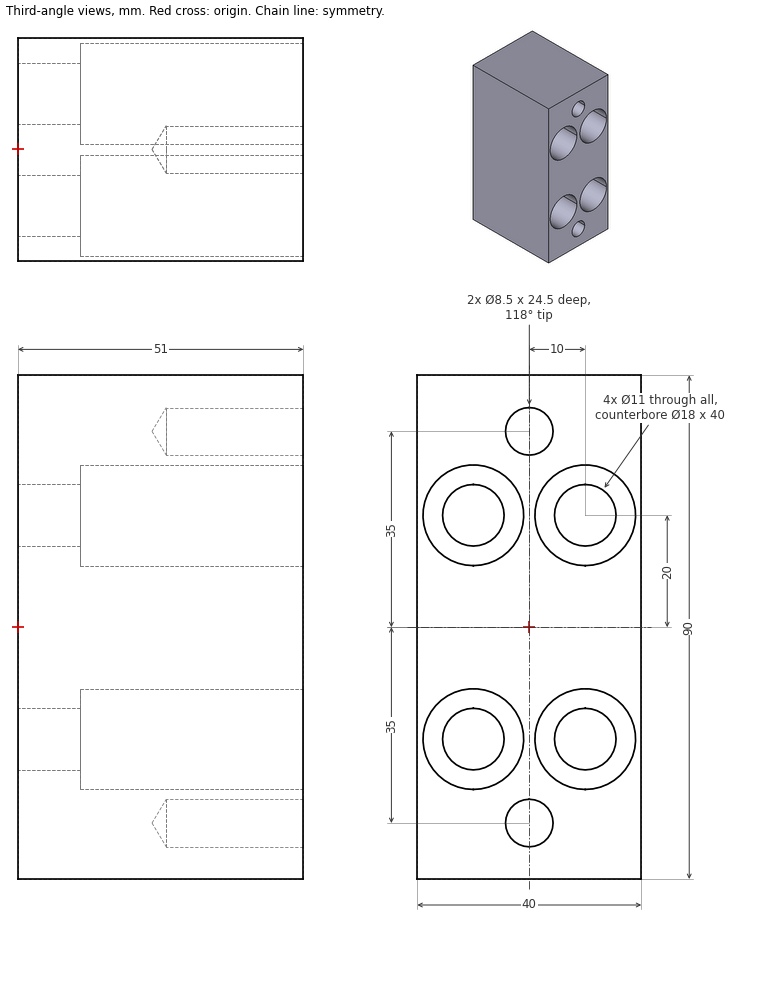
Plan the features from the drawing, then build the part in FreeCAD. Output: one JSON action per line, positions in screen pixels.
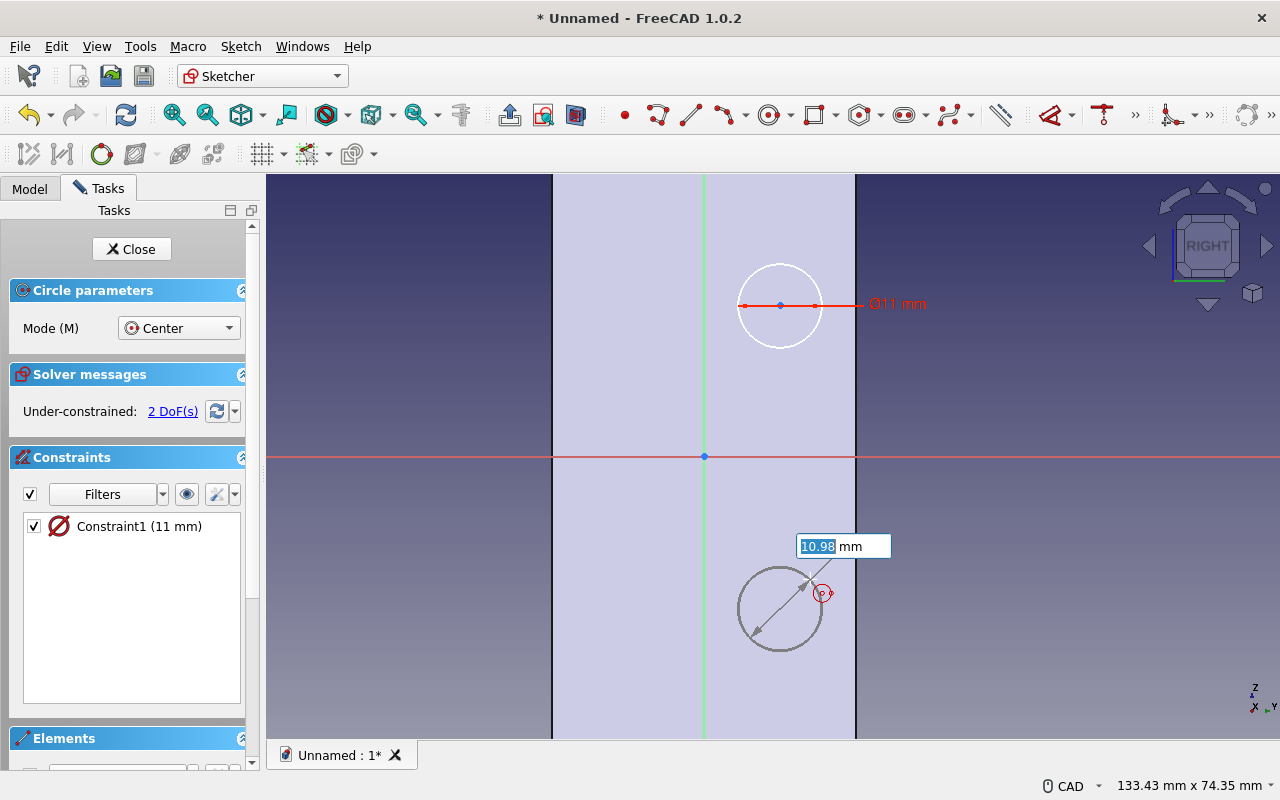
{"action": "type", "text": "11"}
{"action": "key", "text": "Return"}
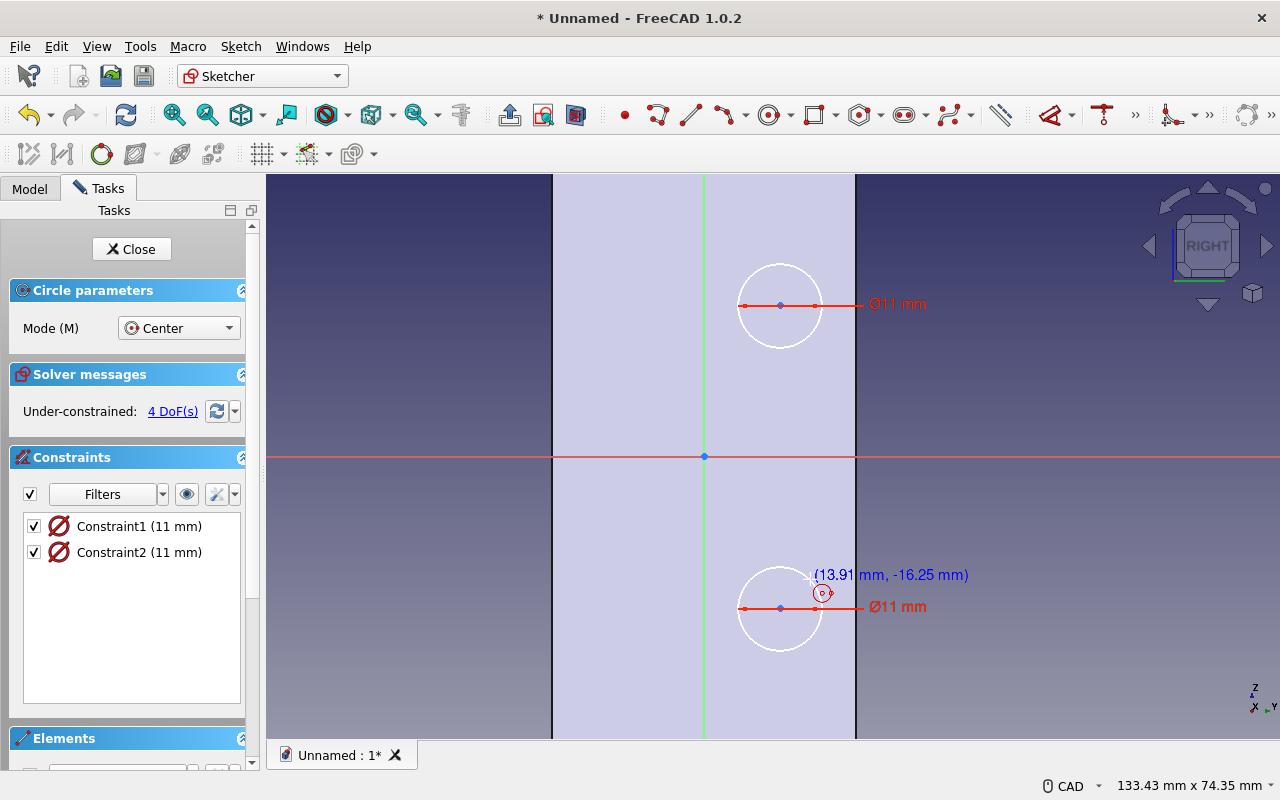
{"action": "left_click", "coordinate": [628, 305]}
{"action": "mouse_move", "coordinate": [658, 275]}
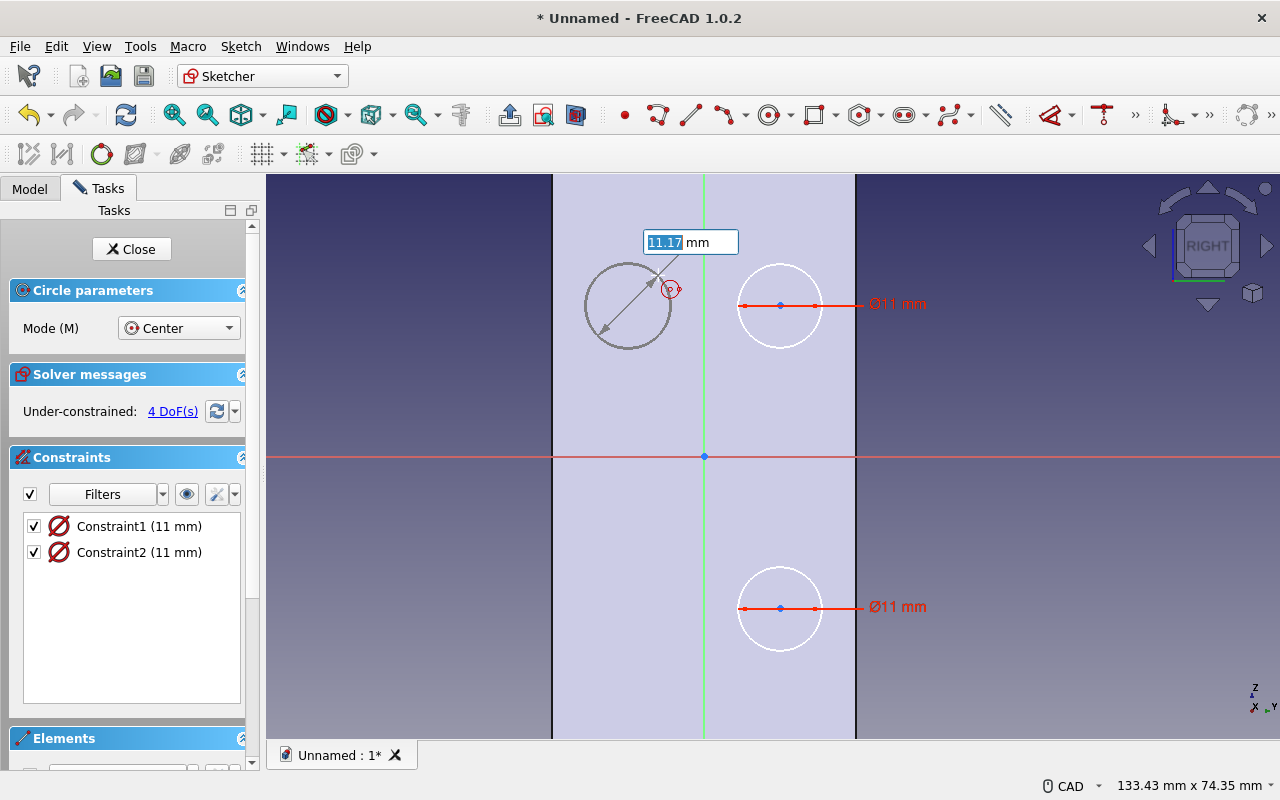
{"action": "type", "text": "11"}
{"action": "key", "text": "Return"}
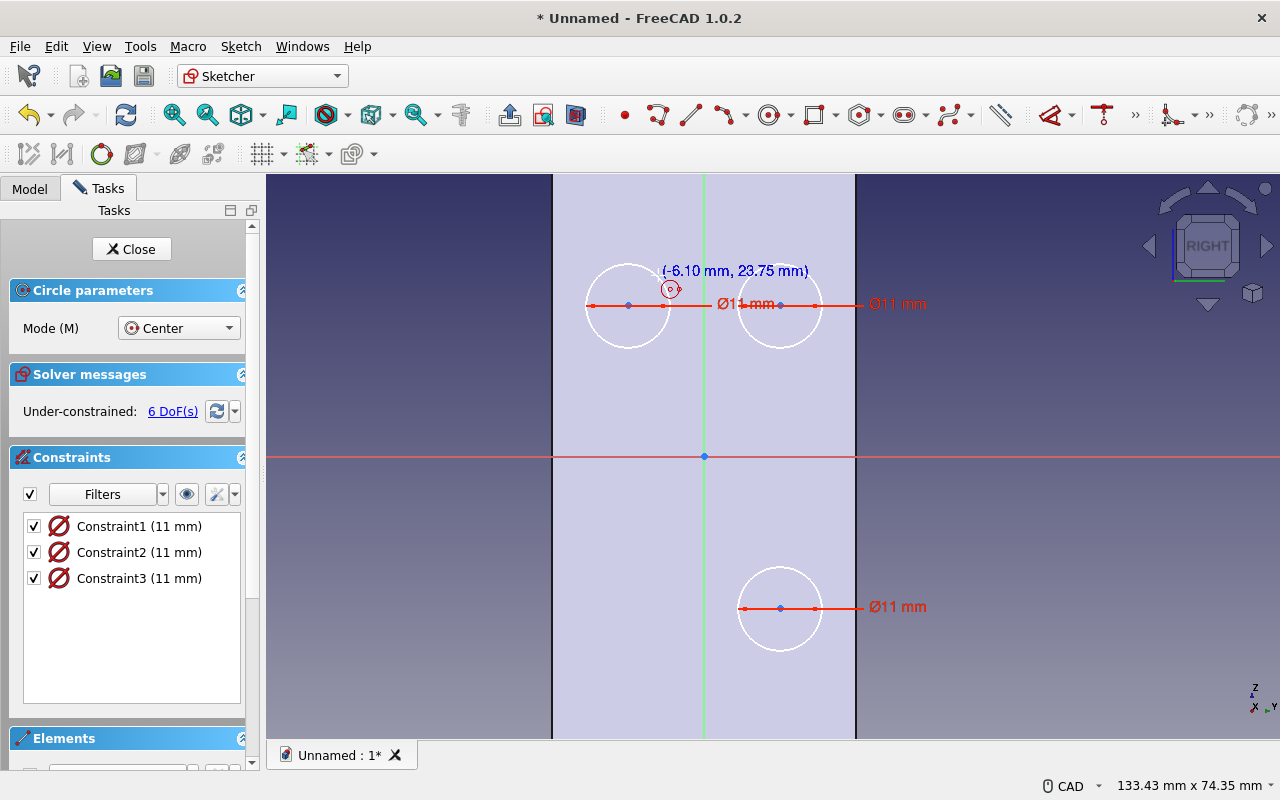
{"action": "left_click", "coordinate": [628, 608]}
{"action": "mouse_move", "coordinate": [658, 579]}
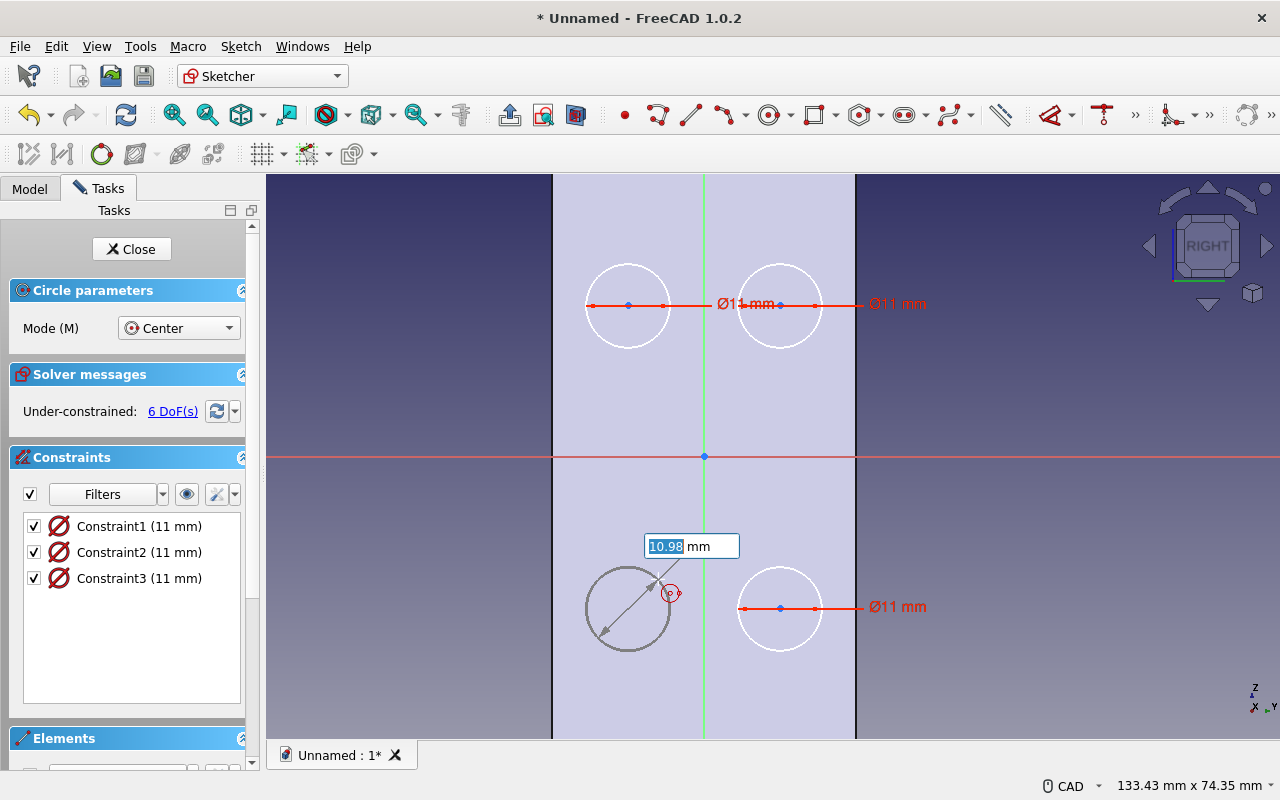
{"action": "type", "text": "11"}
{"action": "key", "text": "Return"}
{"action": "key", "text": "Escape"}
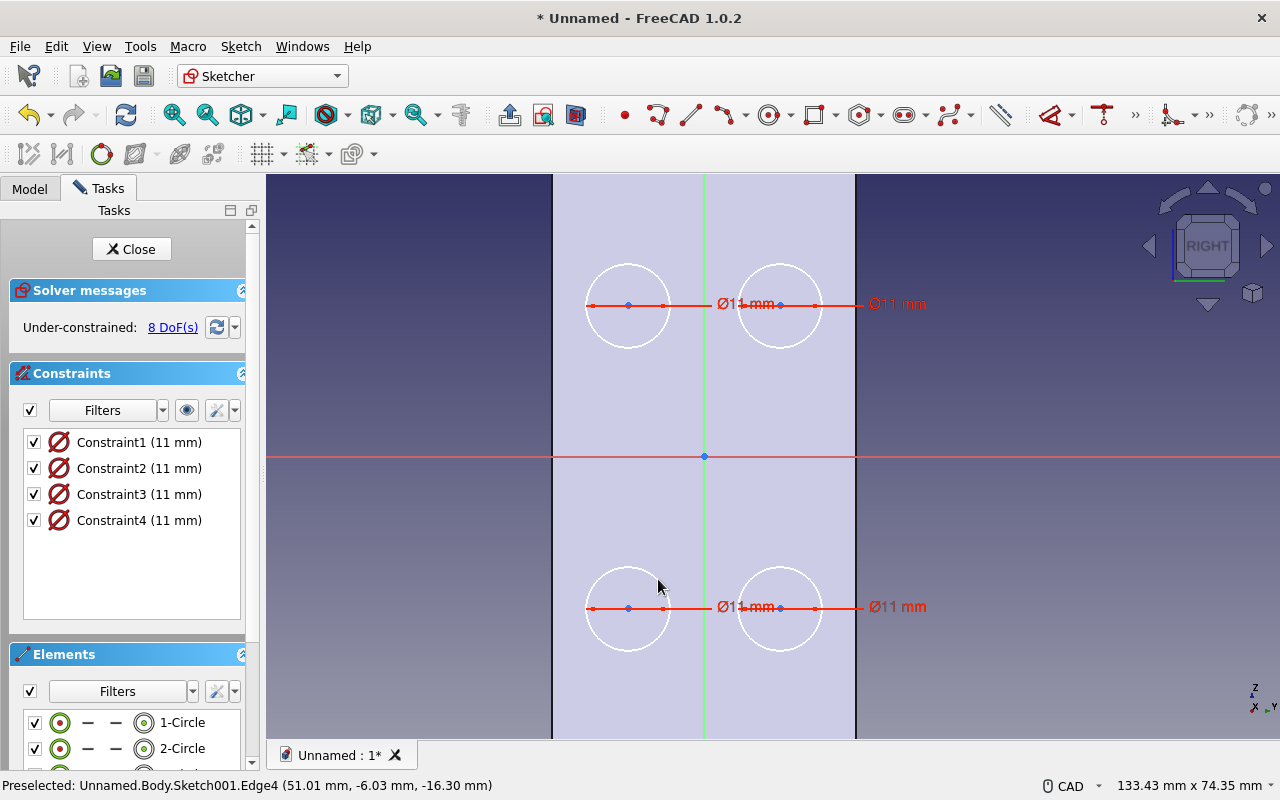
{"action": "left_click", "coordinate": [780, 306]}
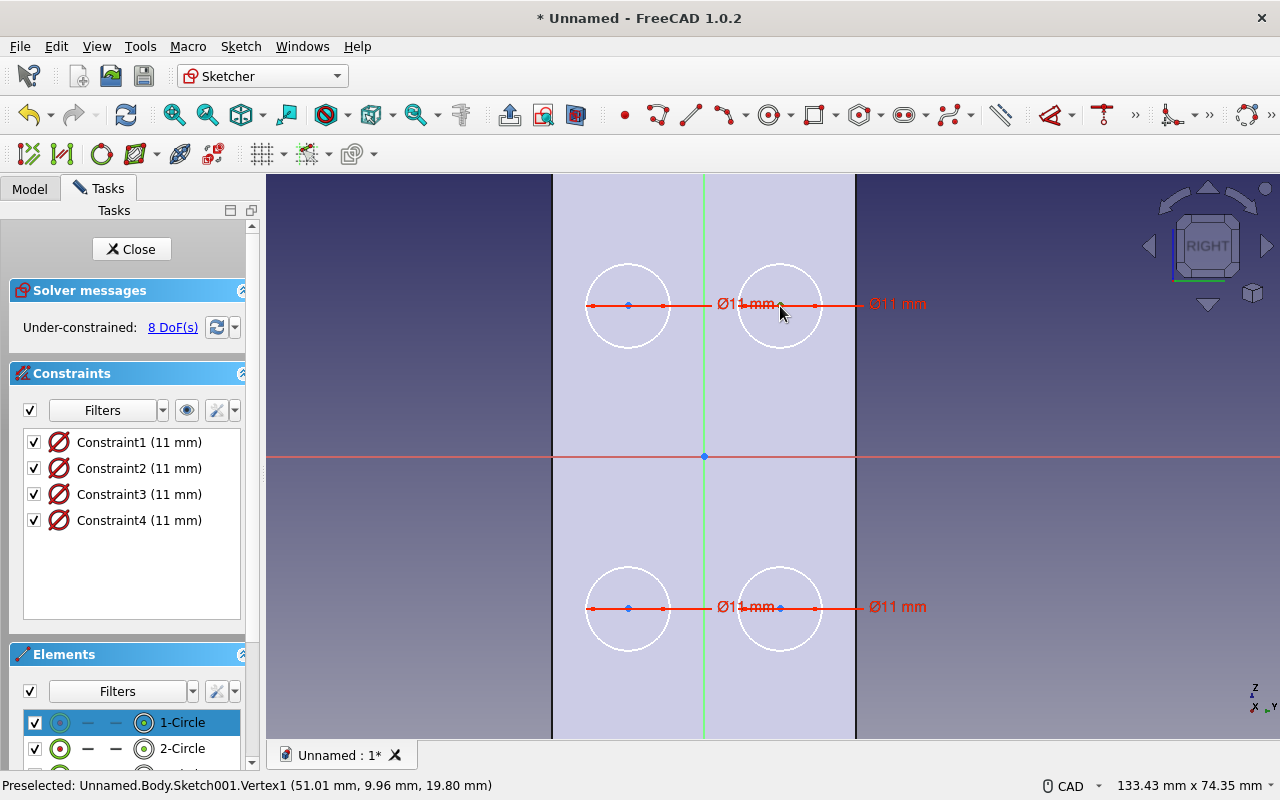
{"action": "left_click", "coordinate": [780, 609]}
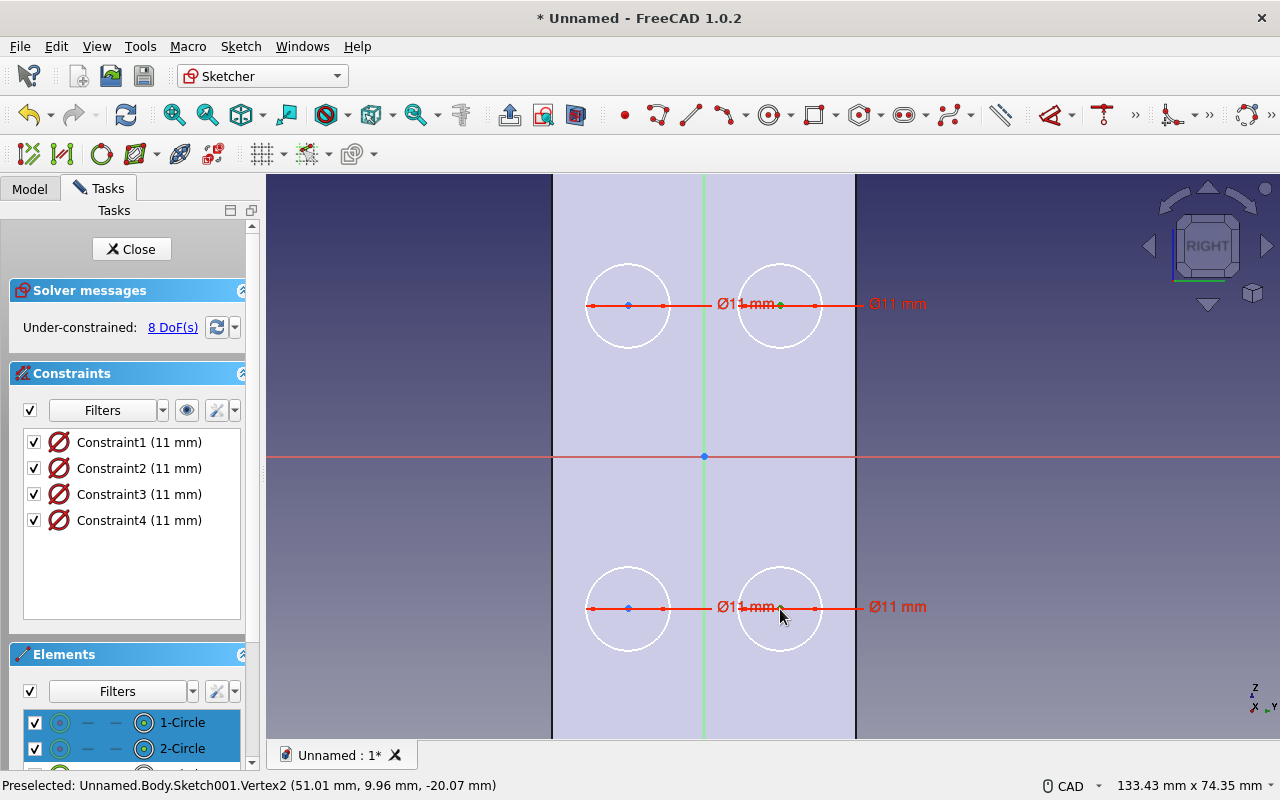
{"action": "left_click", "coordinate": [353, 456]}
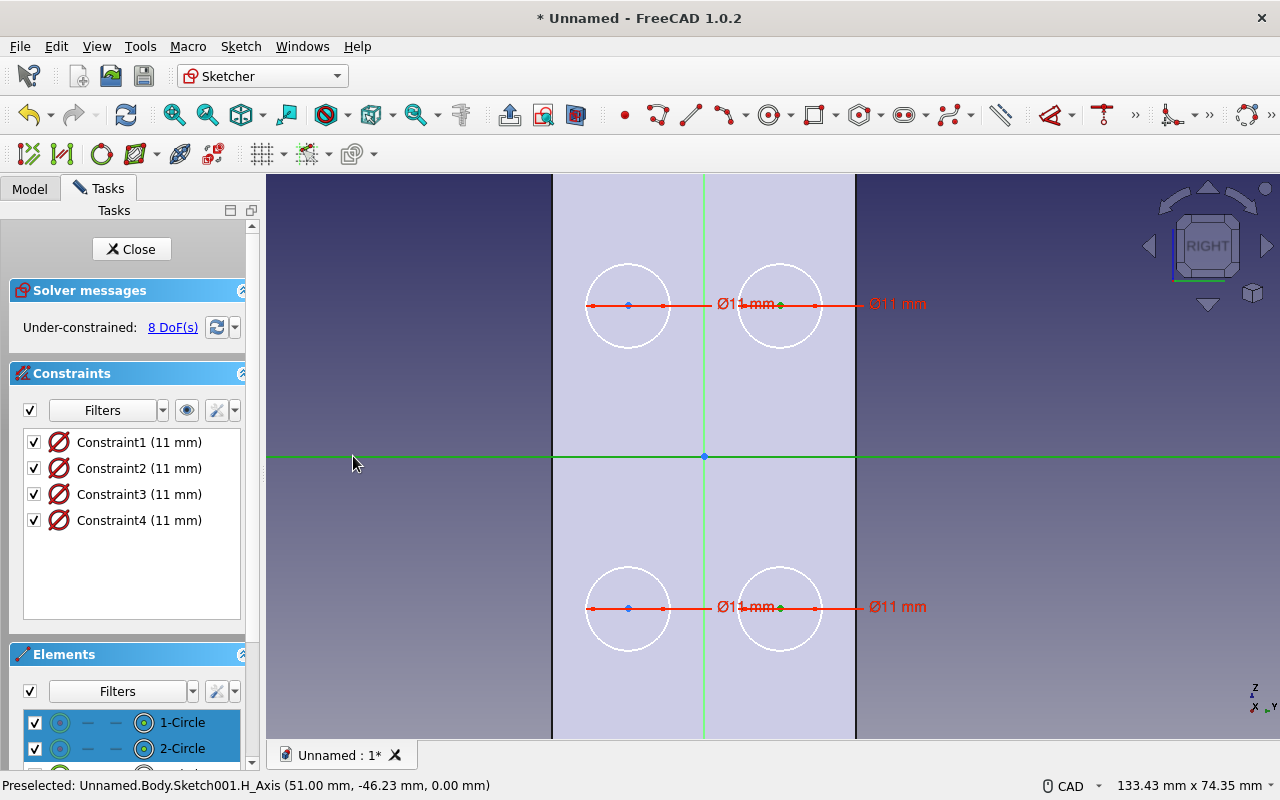
{"action": "key", "text": "s"}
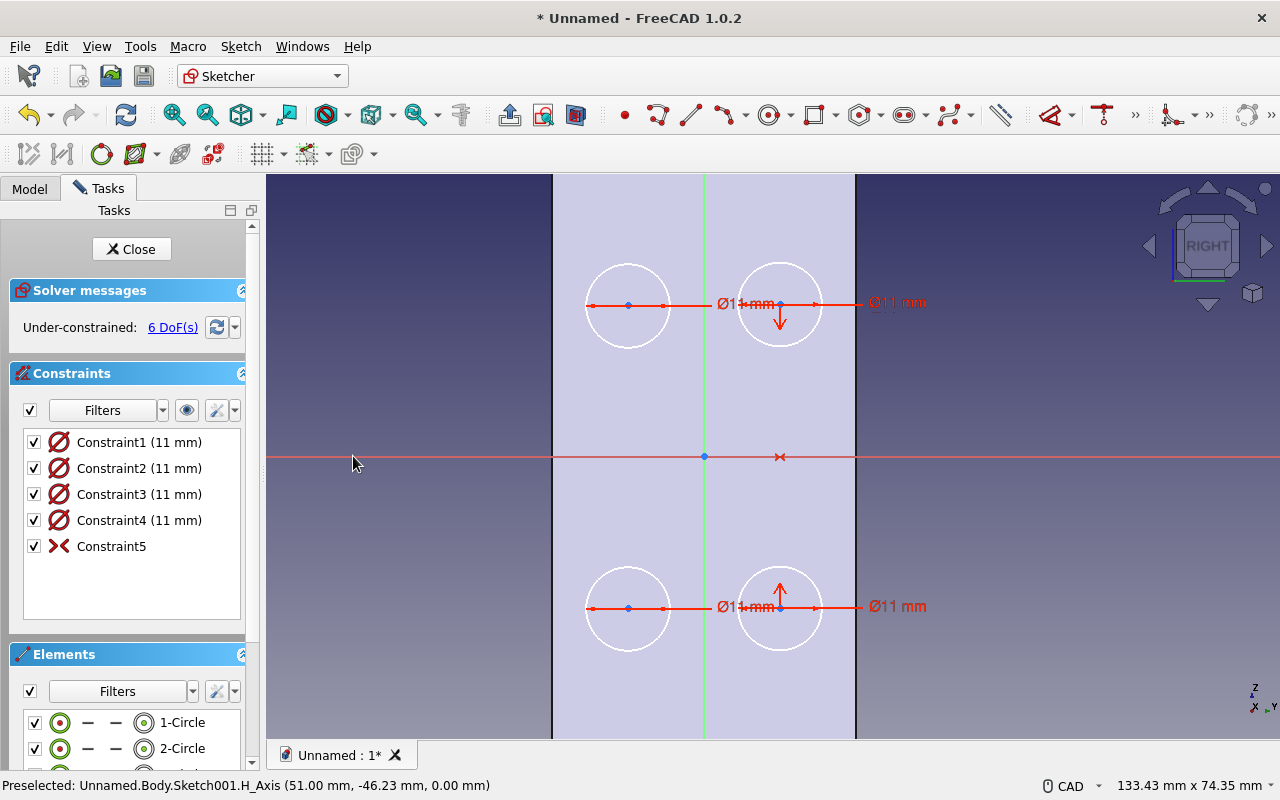
{"action": "left_click", "coordinate": [780, 305]}